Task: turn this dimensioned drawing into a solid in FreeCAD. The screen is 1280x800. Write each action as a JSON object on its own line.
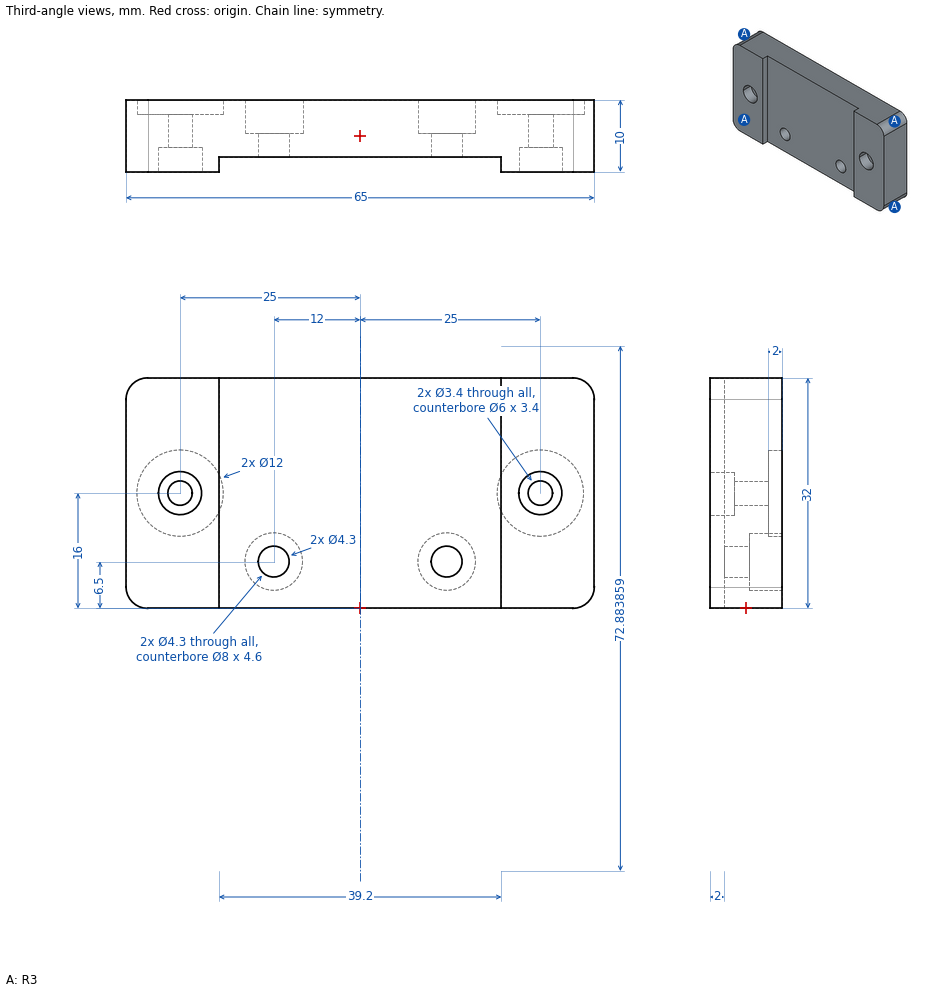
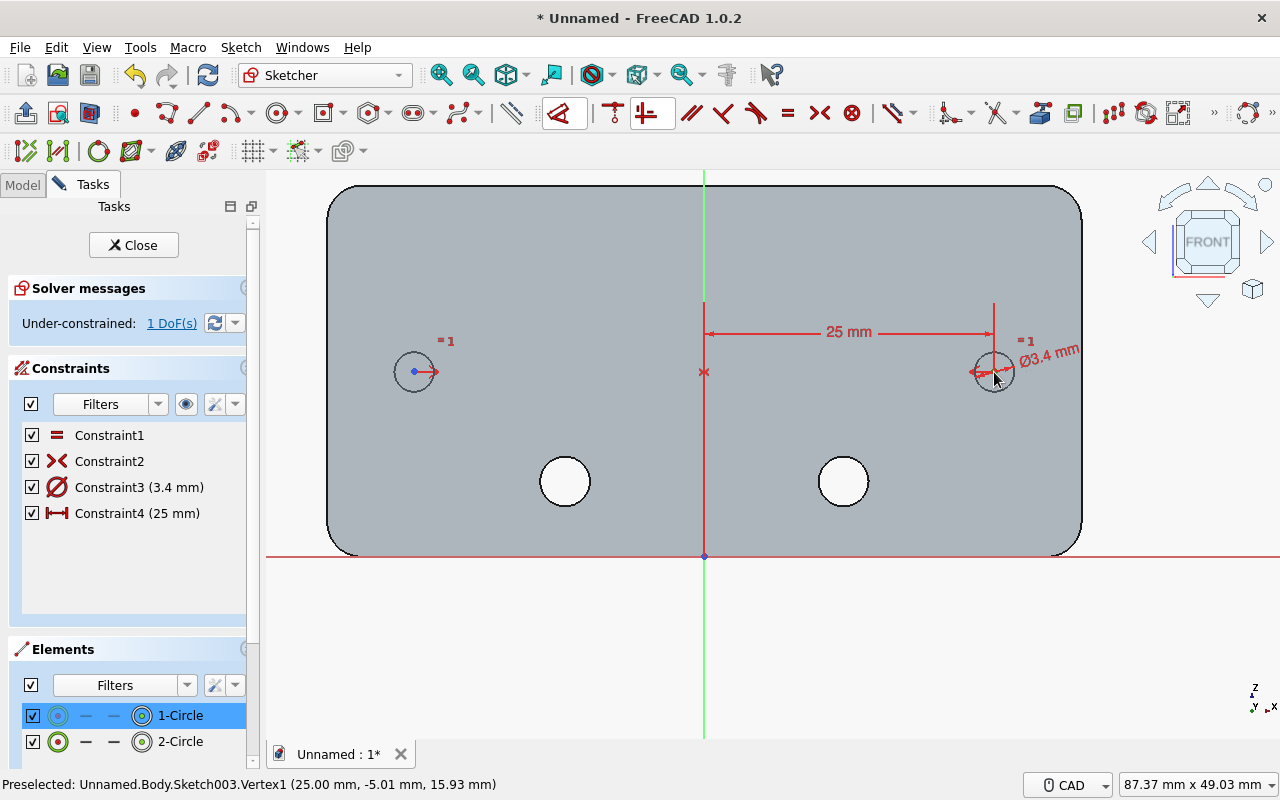
{"action": "left_click", "coordinate": [582, 114]}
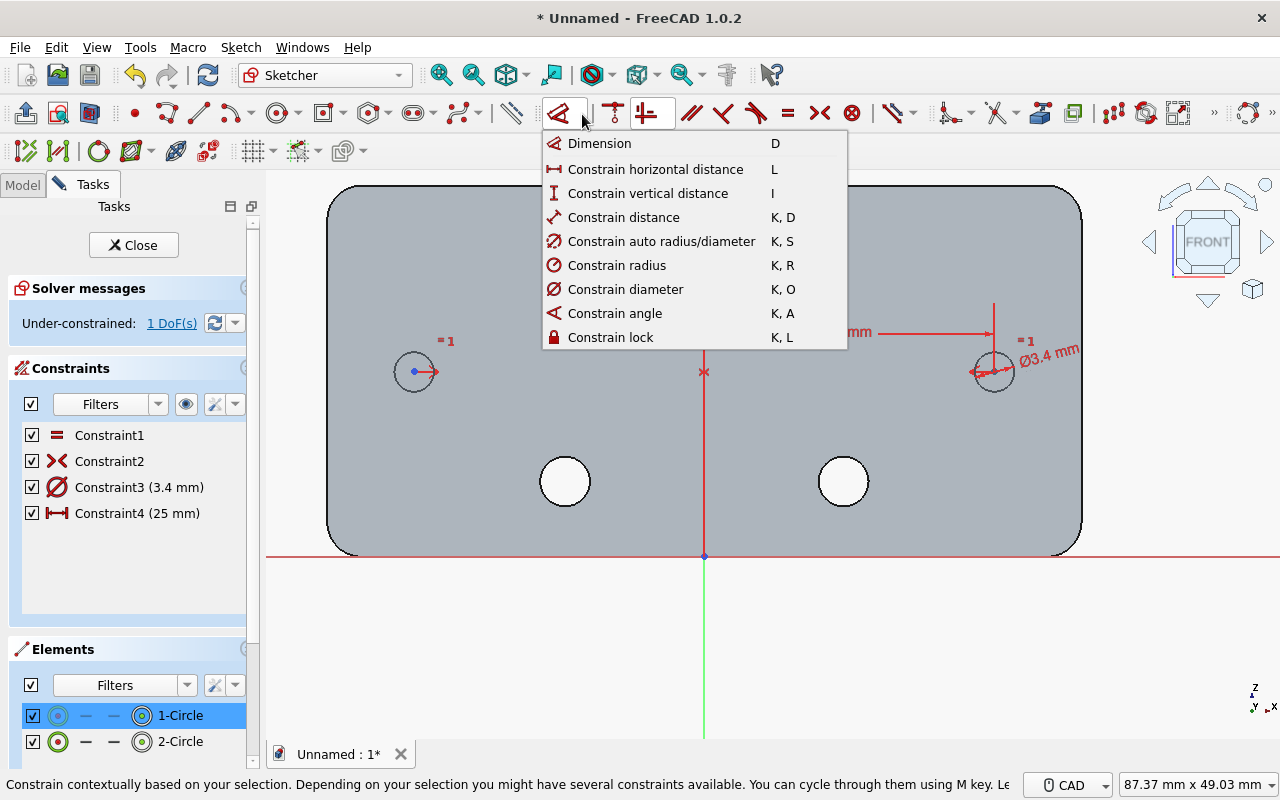
{"action": "left_click", "coordinate": [695, 193]}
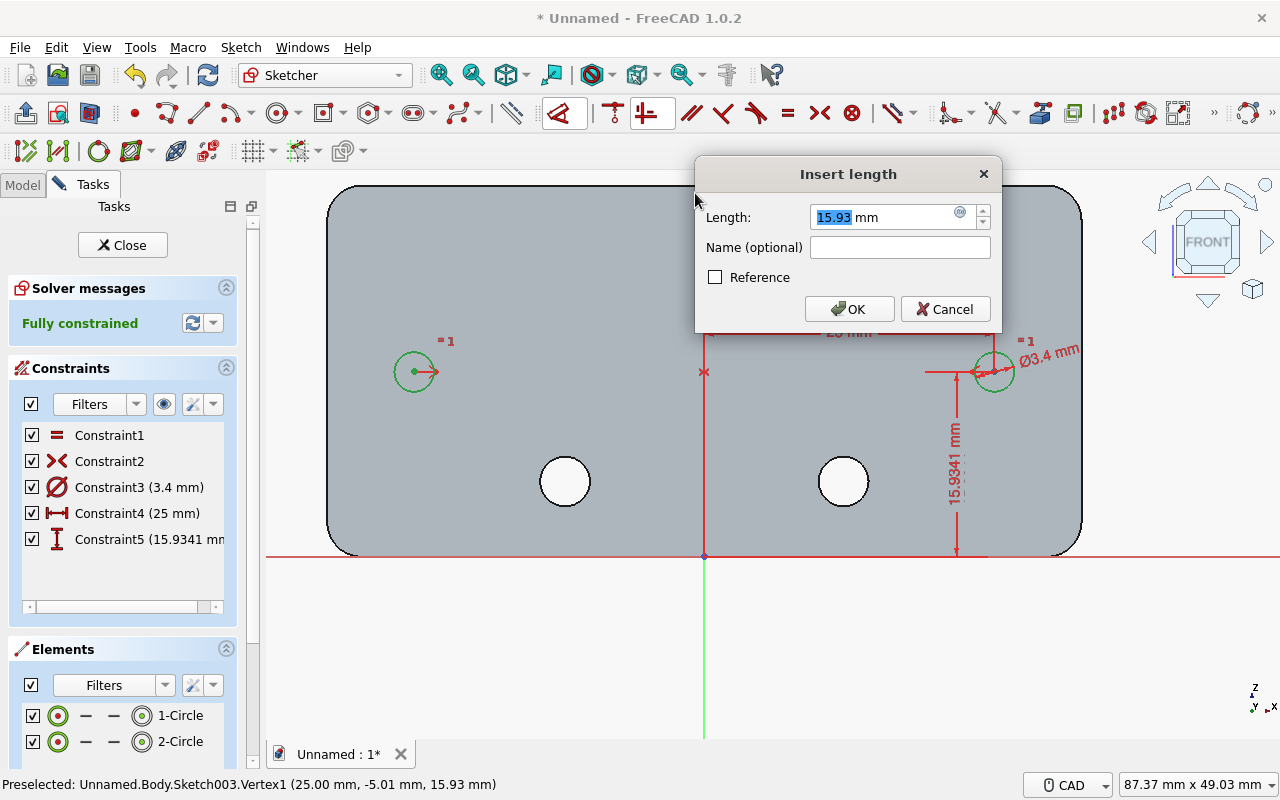
{"action": "type", "text": "16"}
{"action": "key", "text": "Return"}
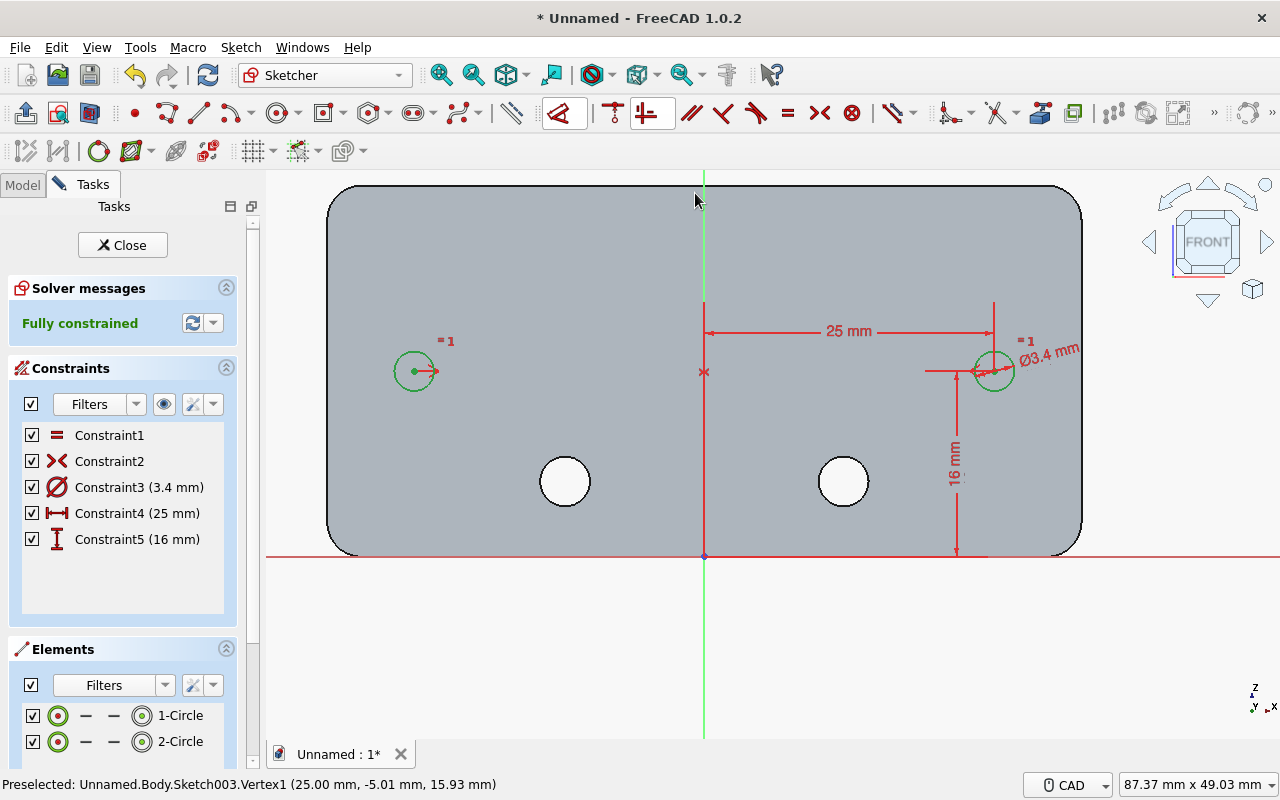
{"action": "left_click", "coordinate": [123, 245]}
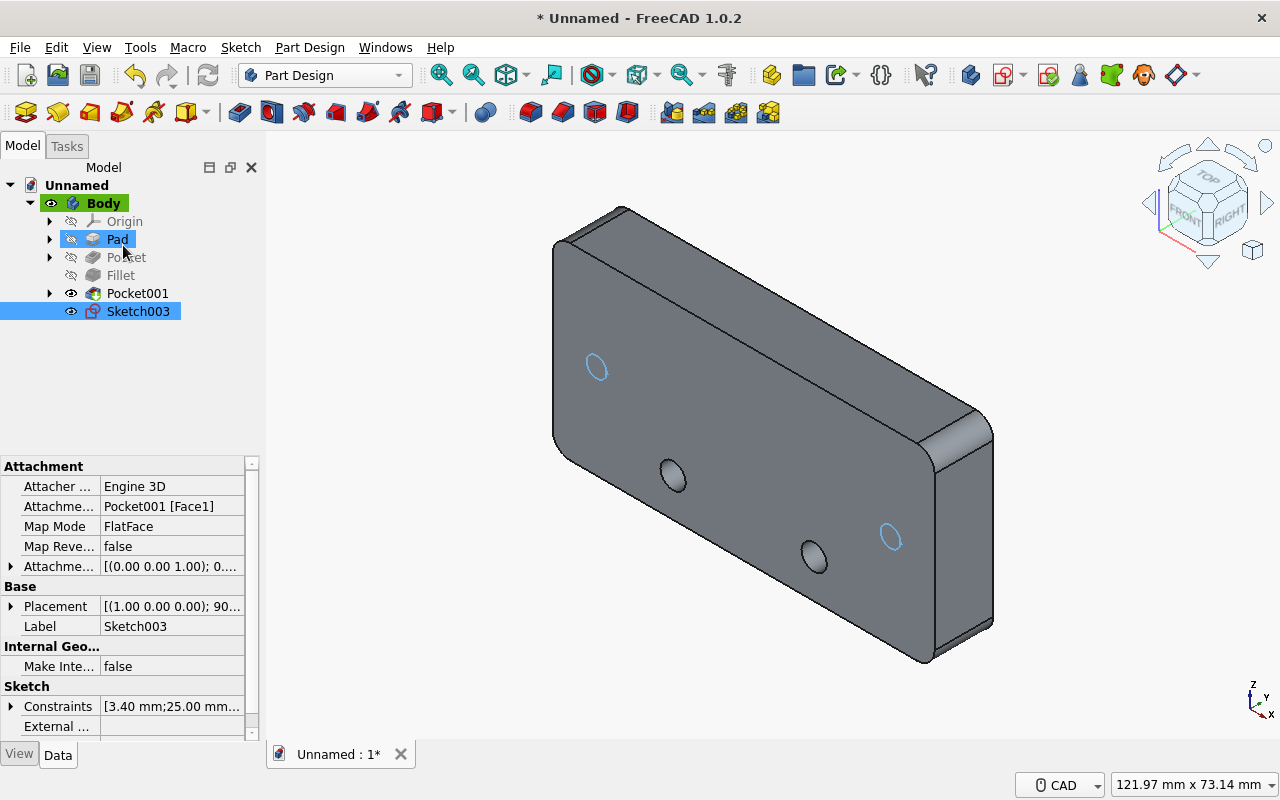
{"action": "left_click", "coordinate": [272, 112]}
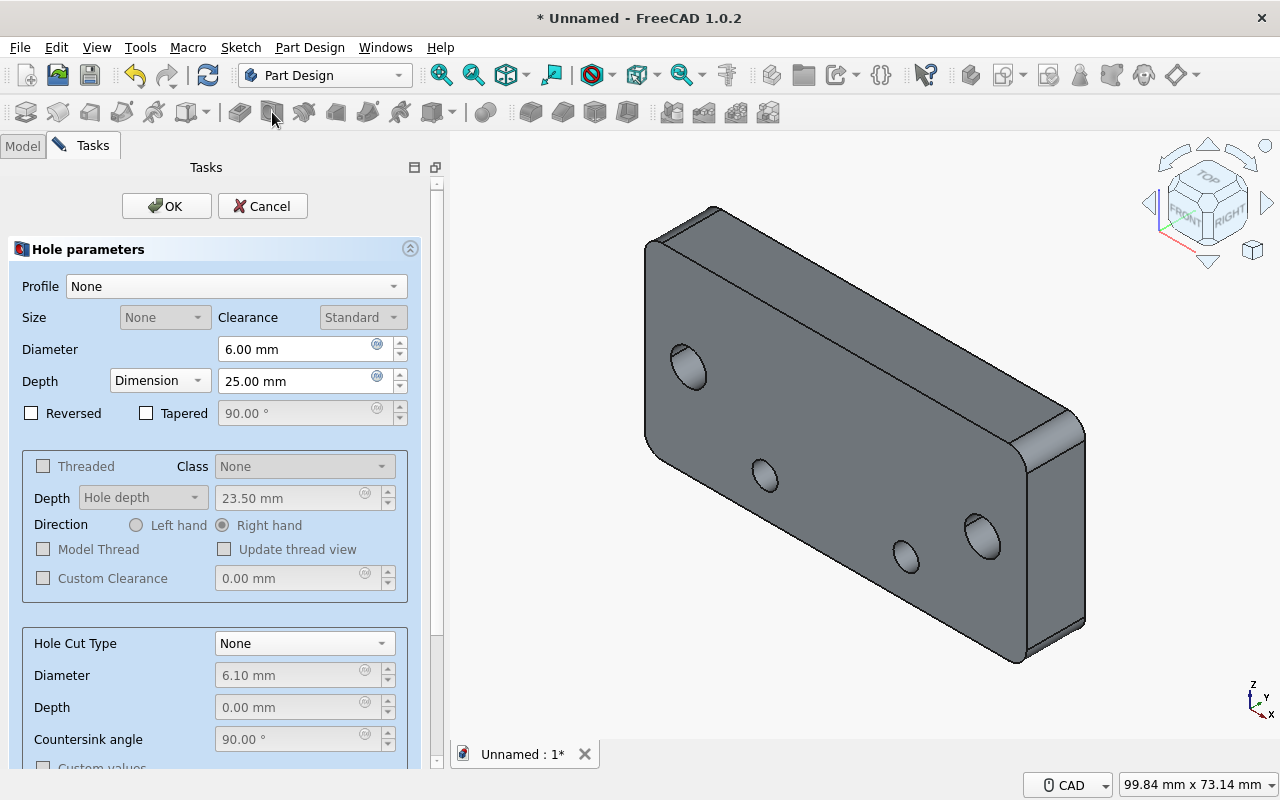
{"action": "triple_click", "coordinate": [305, 349]}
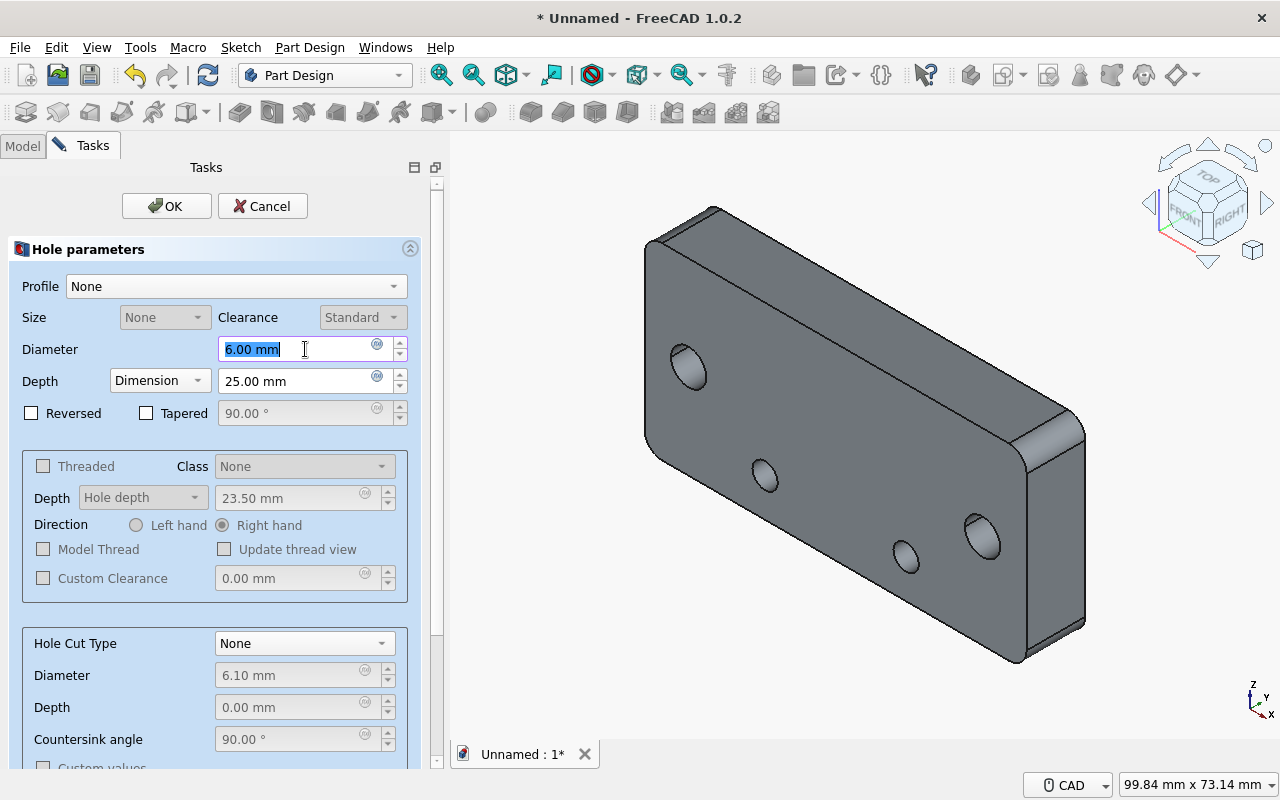
{"action": "type", "text": "3.4"}
{"action": "key", "text": "Tab"}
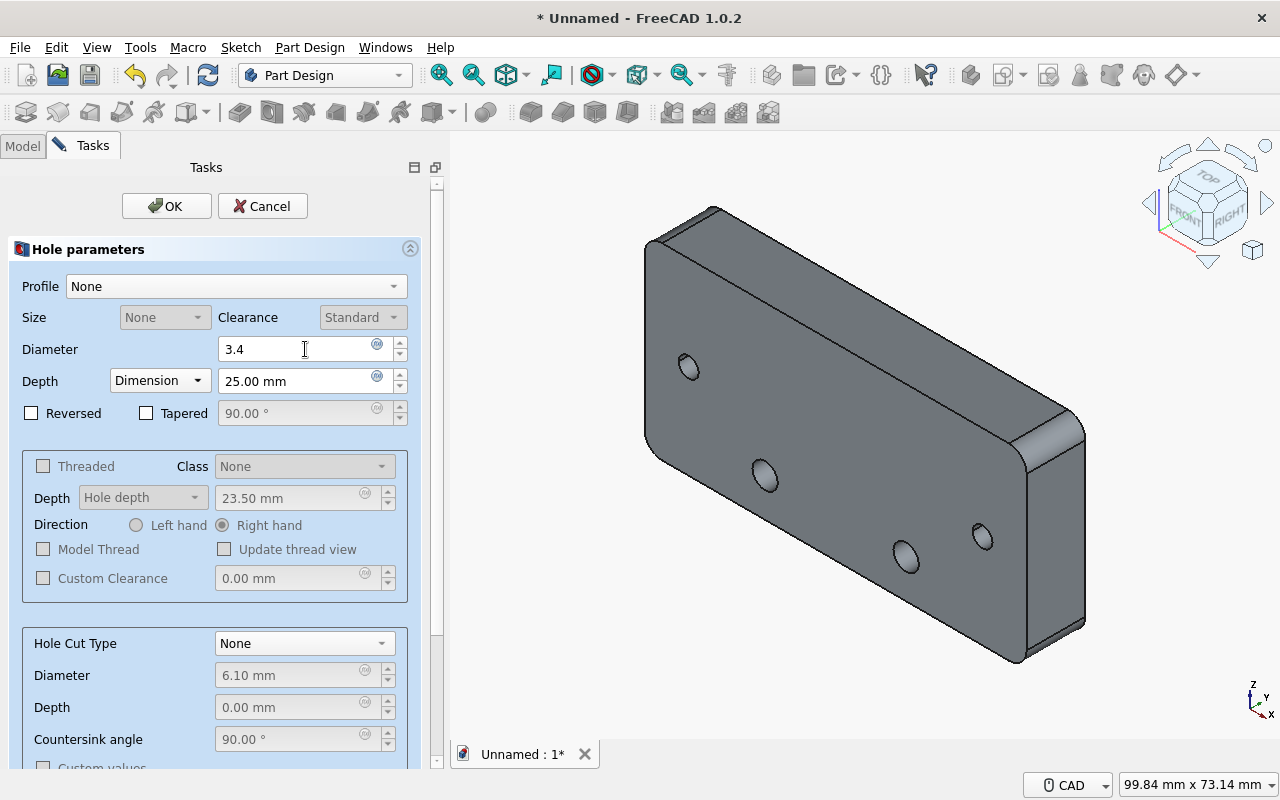
{"action": "left_click", "coordinate": [161, 380]}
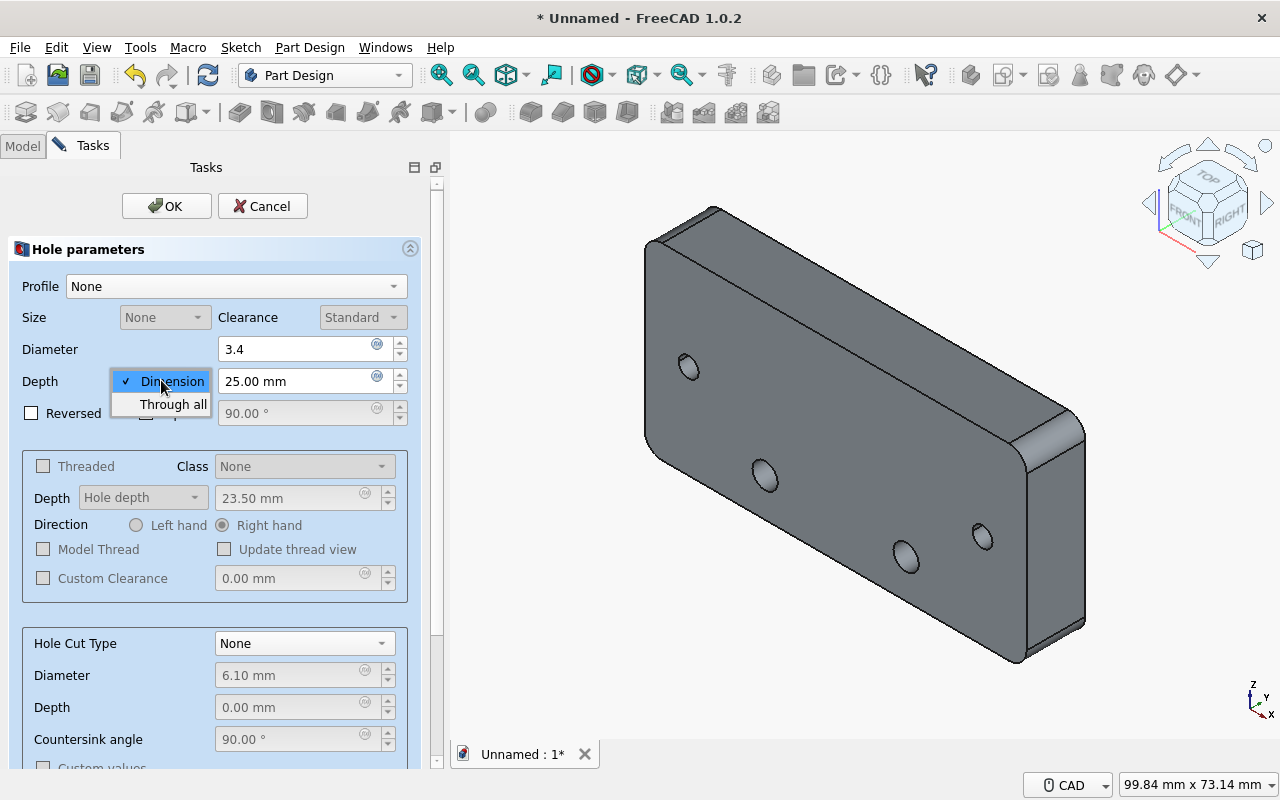
{"action": "left_click", "coordinate": [160, 404]}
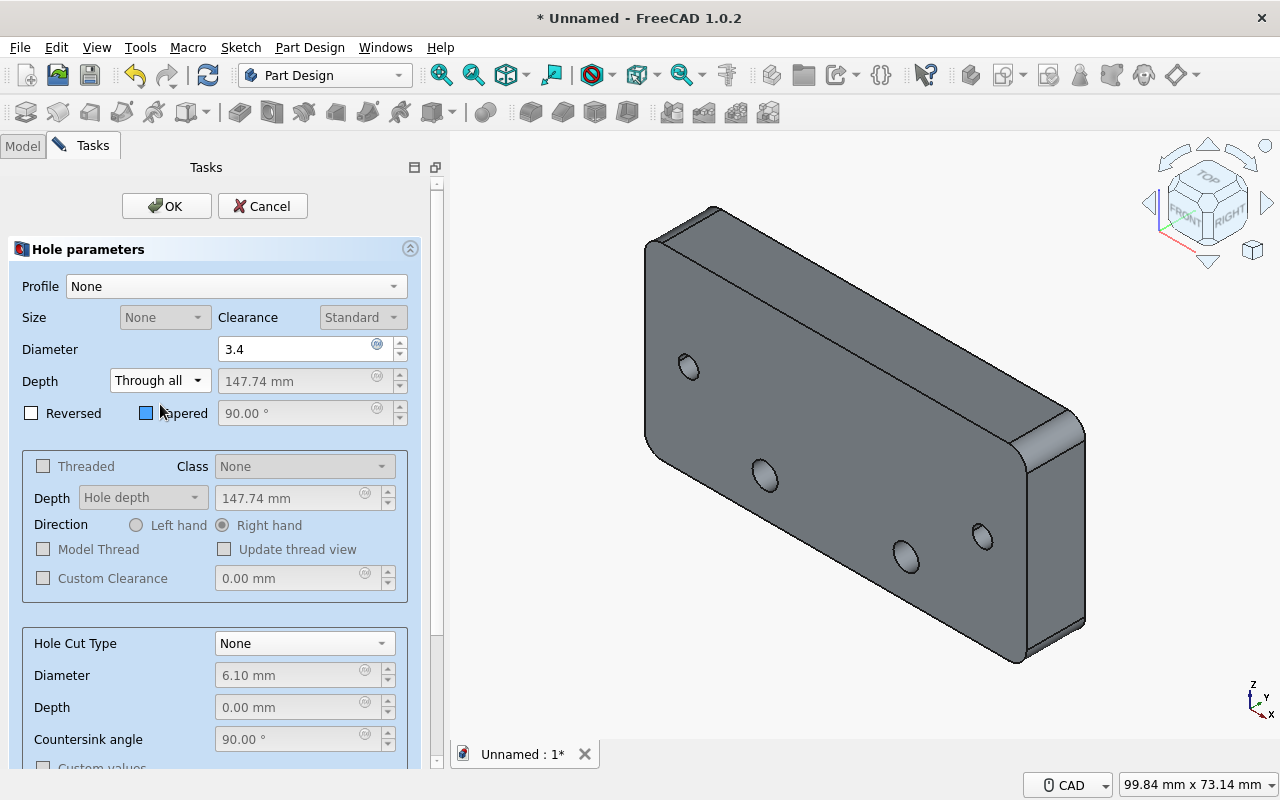
{"action": "left_click", "coordinate": [306, 644]}